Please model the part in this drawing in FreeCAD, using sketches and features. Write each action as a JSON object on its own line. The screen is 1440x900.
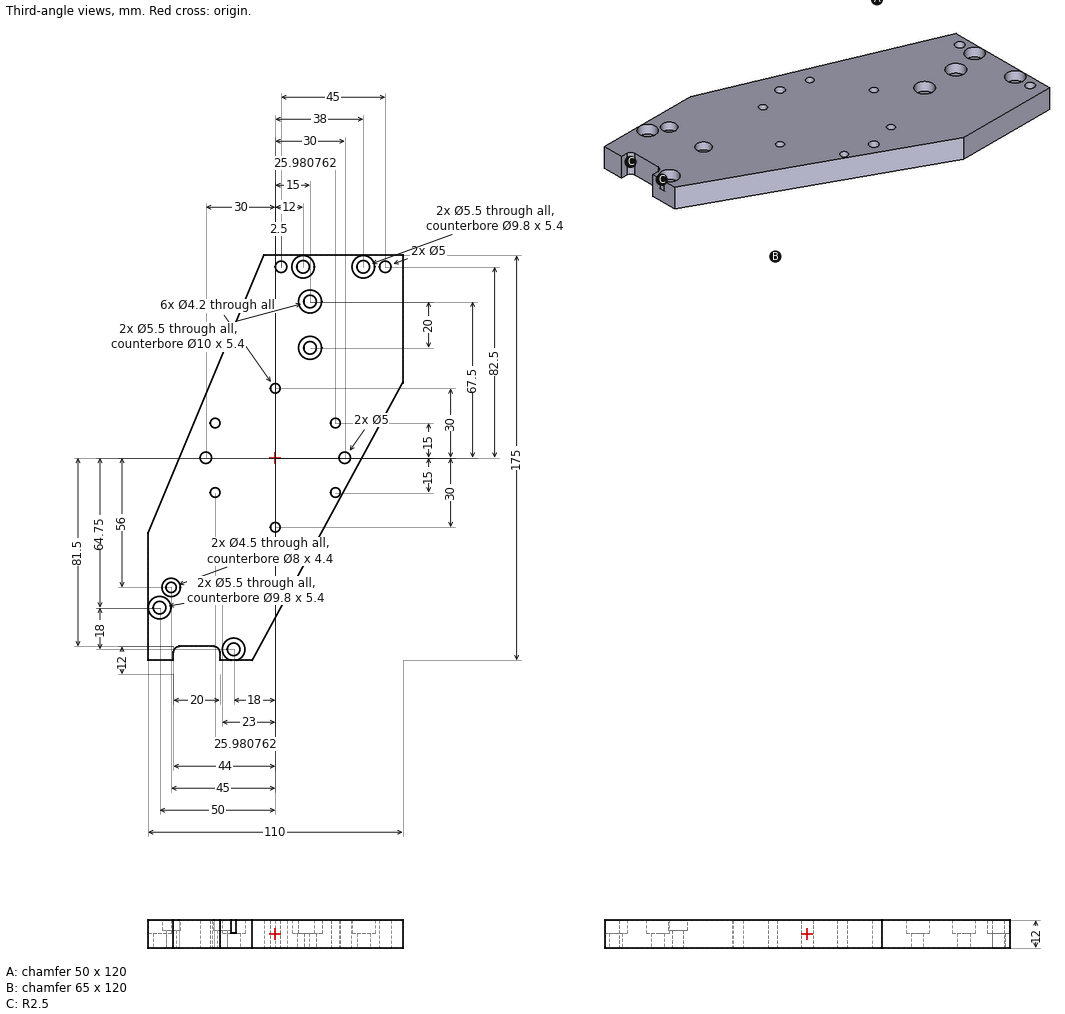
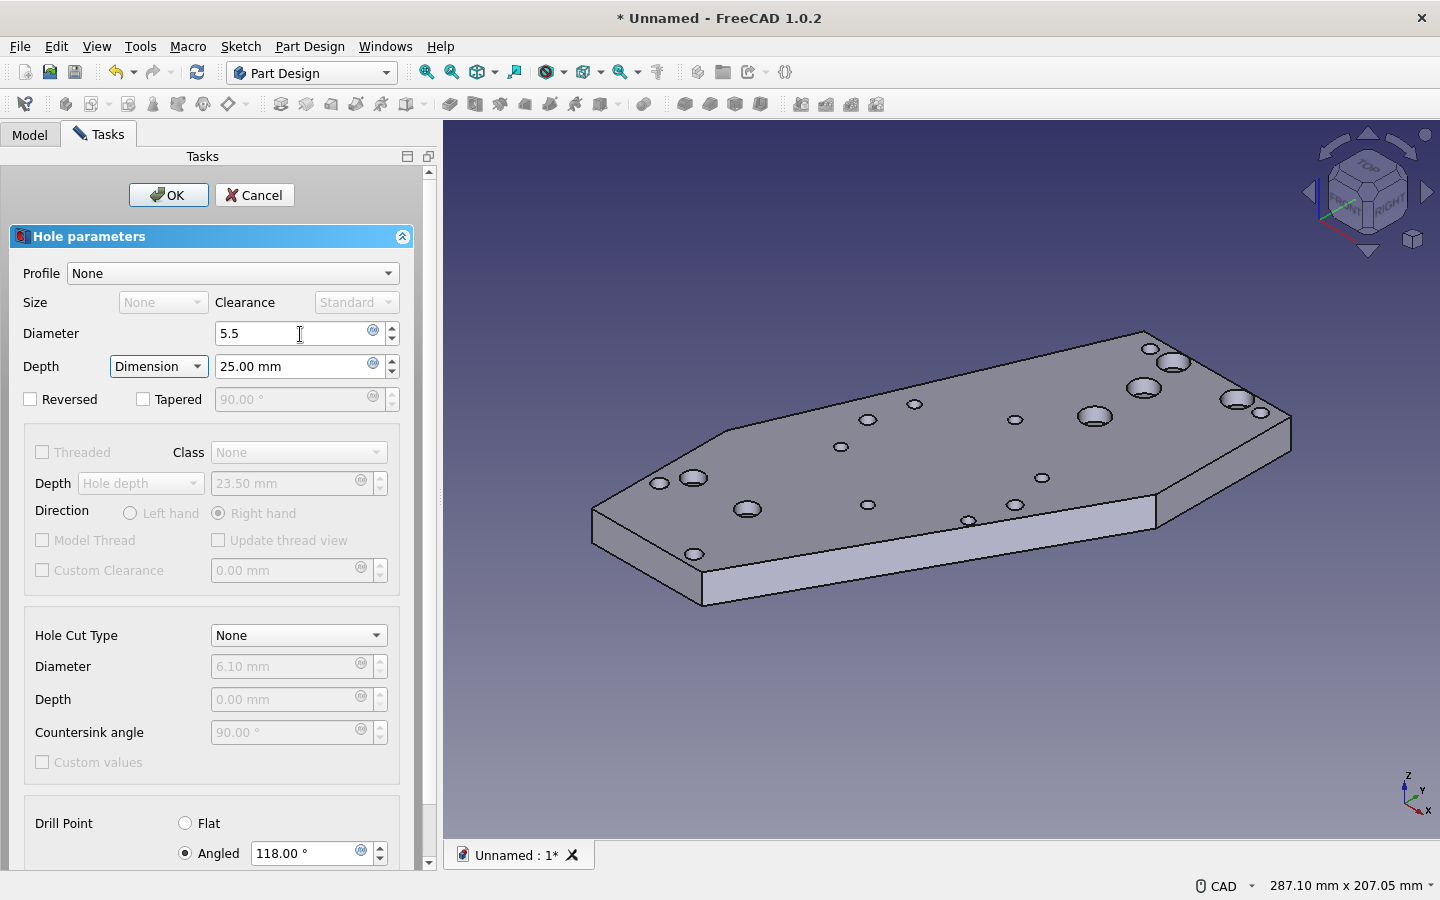
{"action": "left_click", "coordinate": [160, 366]}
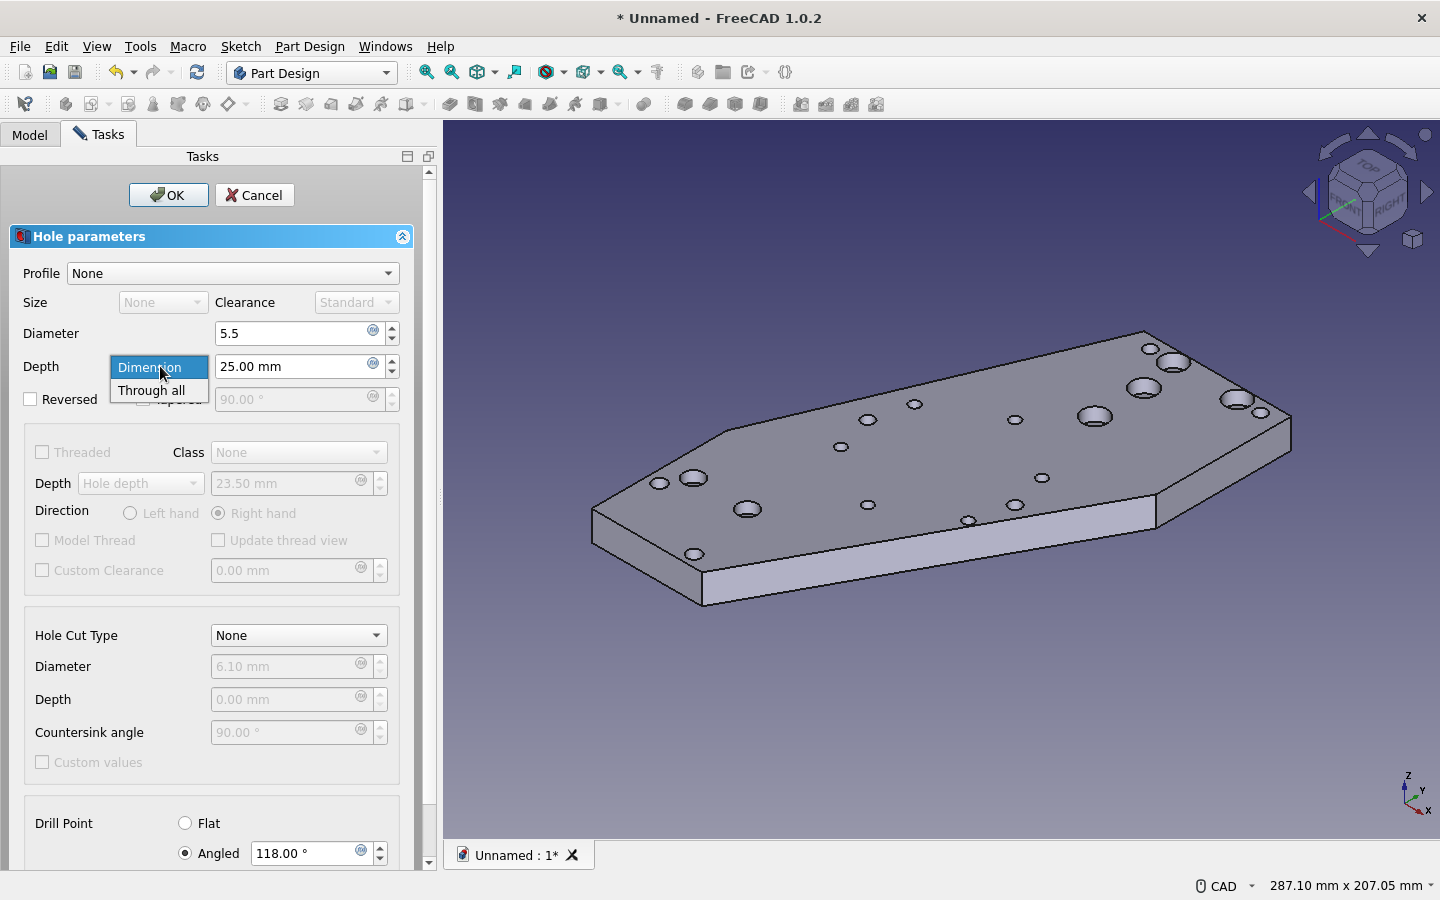
{"action": "left_click", "coordinate": [158, 390]}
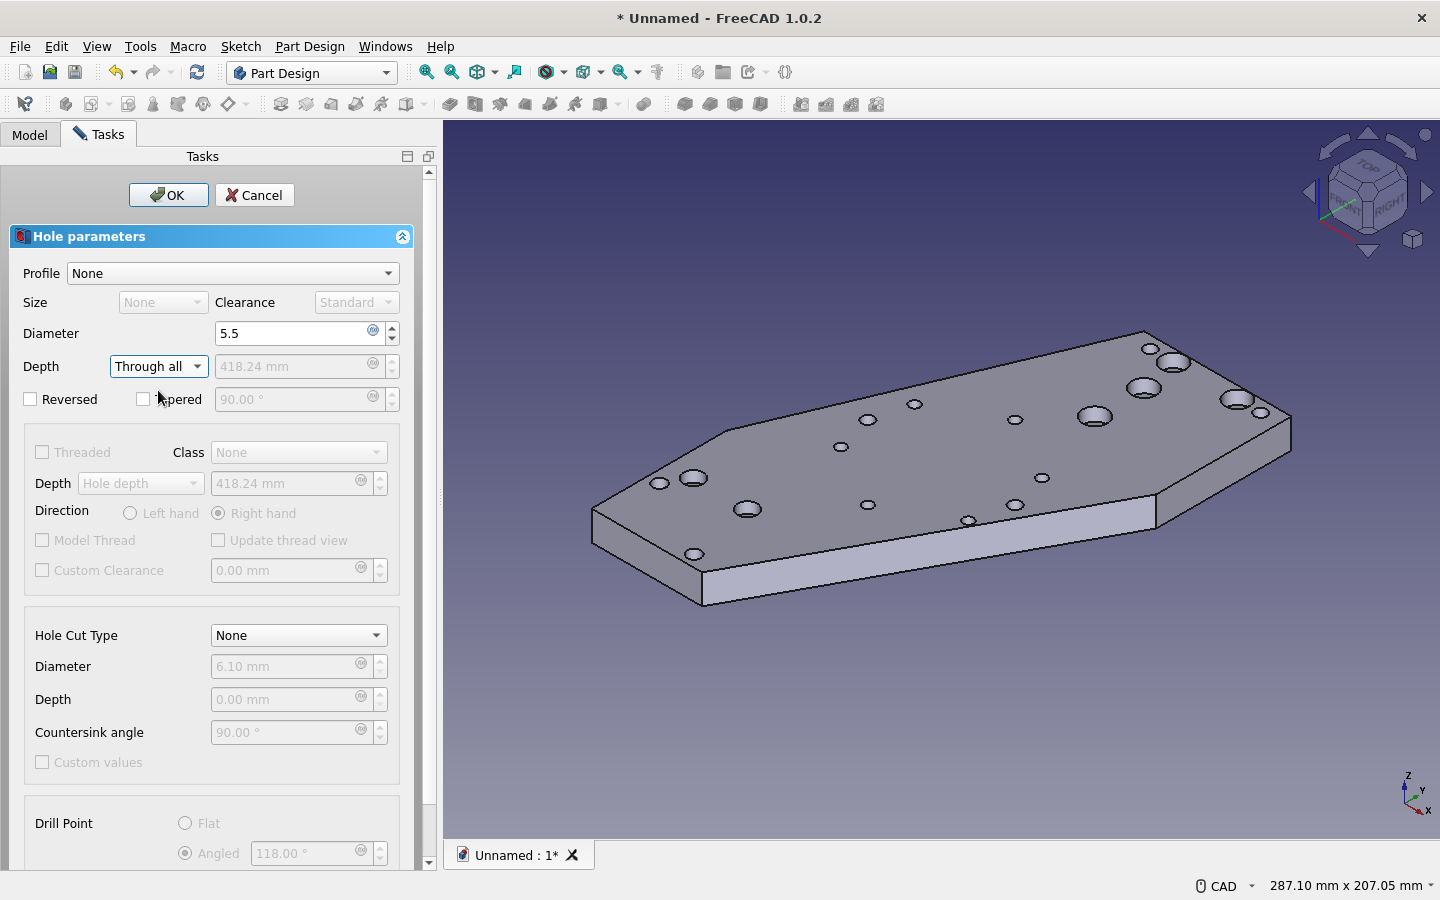
{"action": "left_click", "coordinate": [300, 636]}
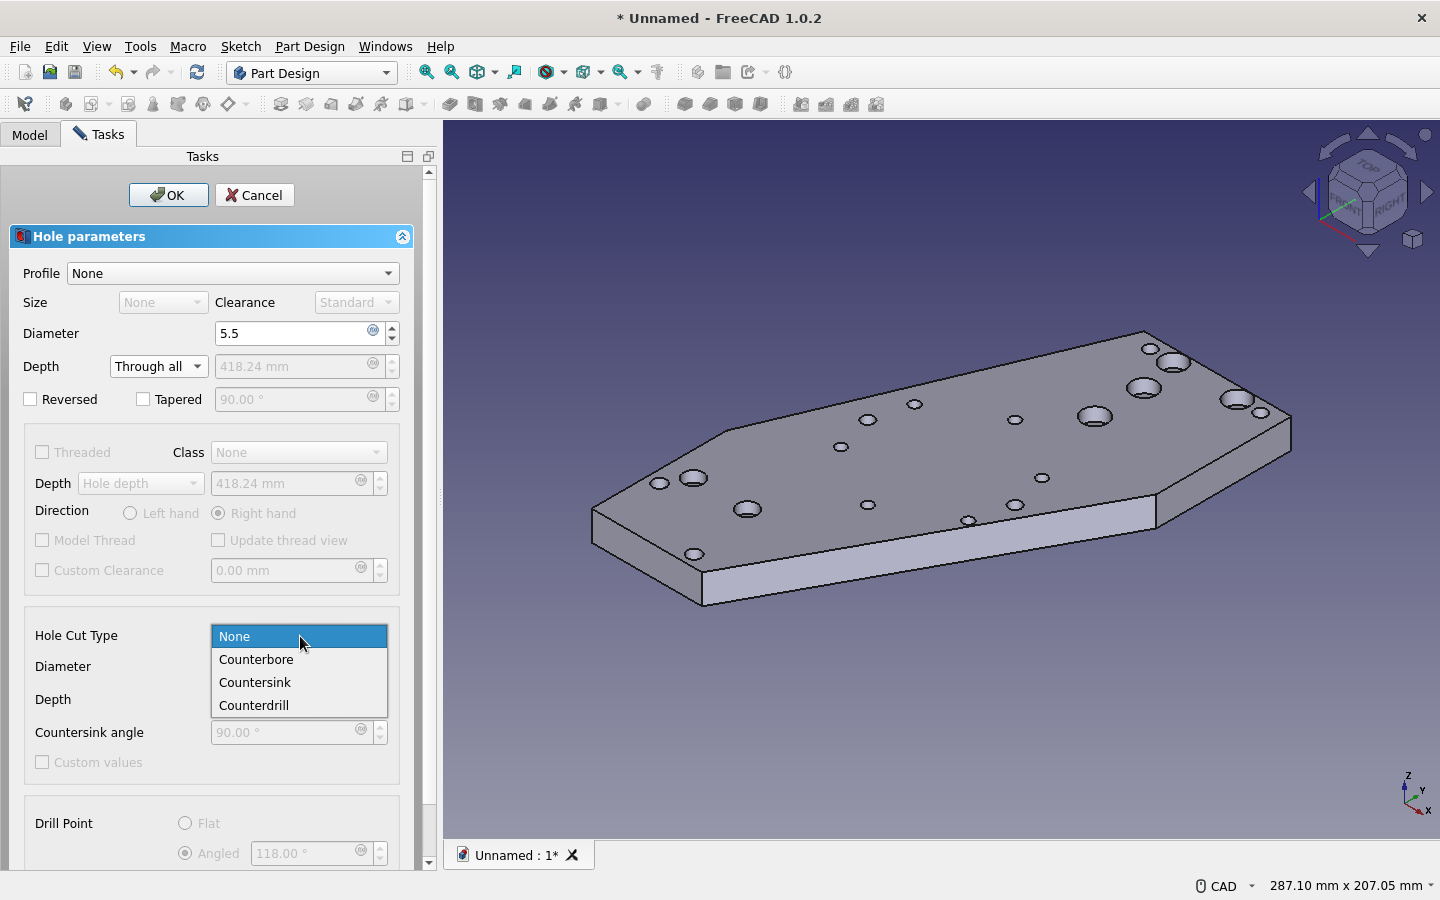
{"action": "left_click", "coordinate": [298, 660]}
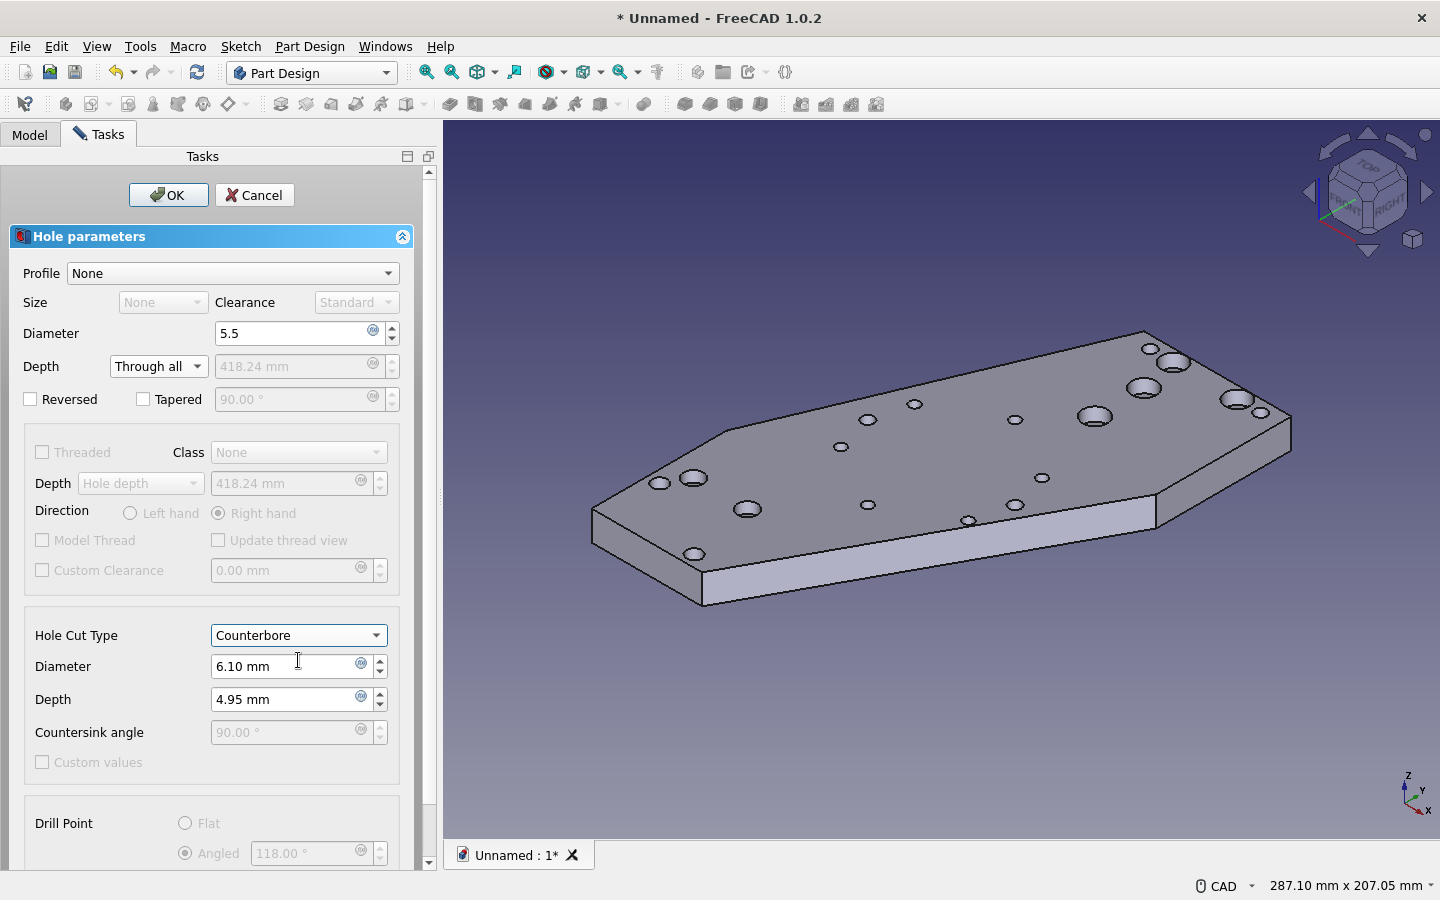
{"action": "triple_click", "coordinate": [292, 666]}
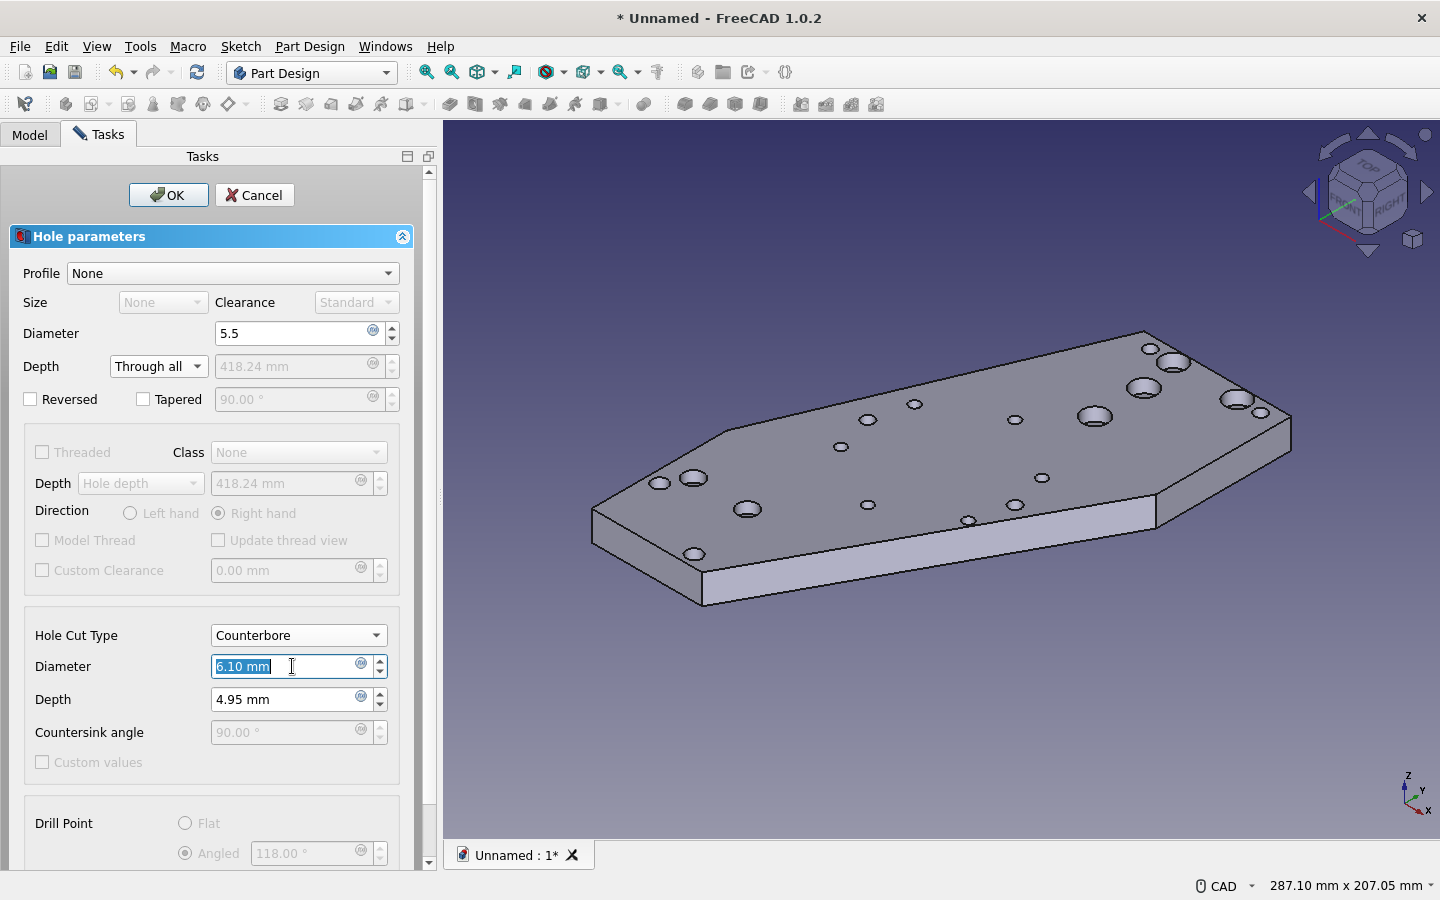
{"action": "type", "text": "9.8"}
{"action": "key", "text": "Tab"}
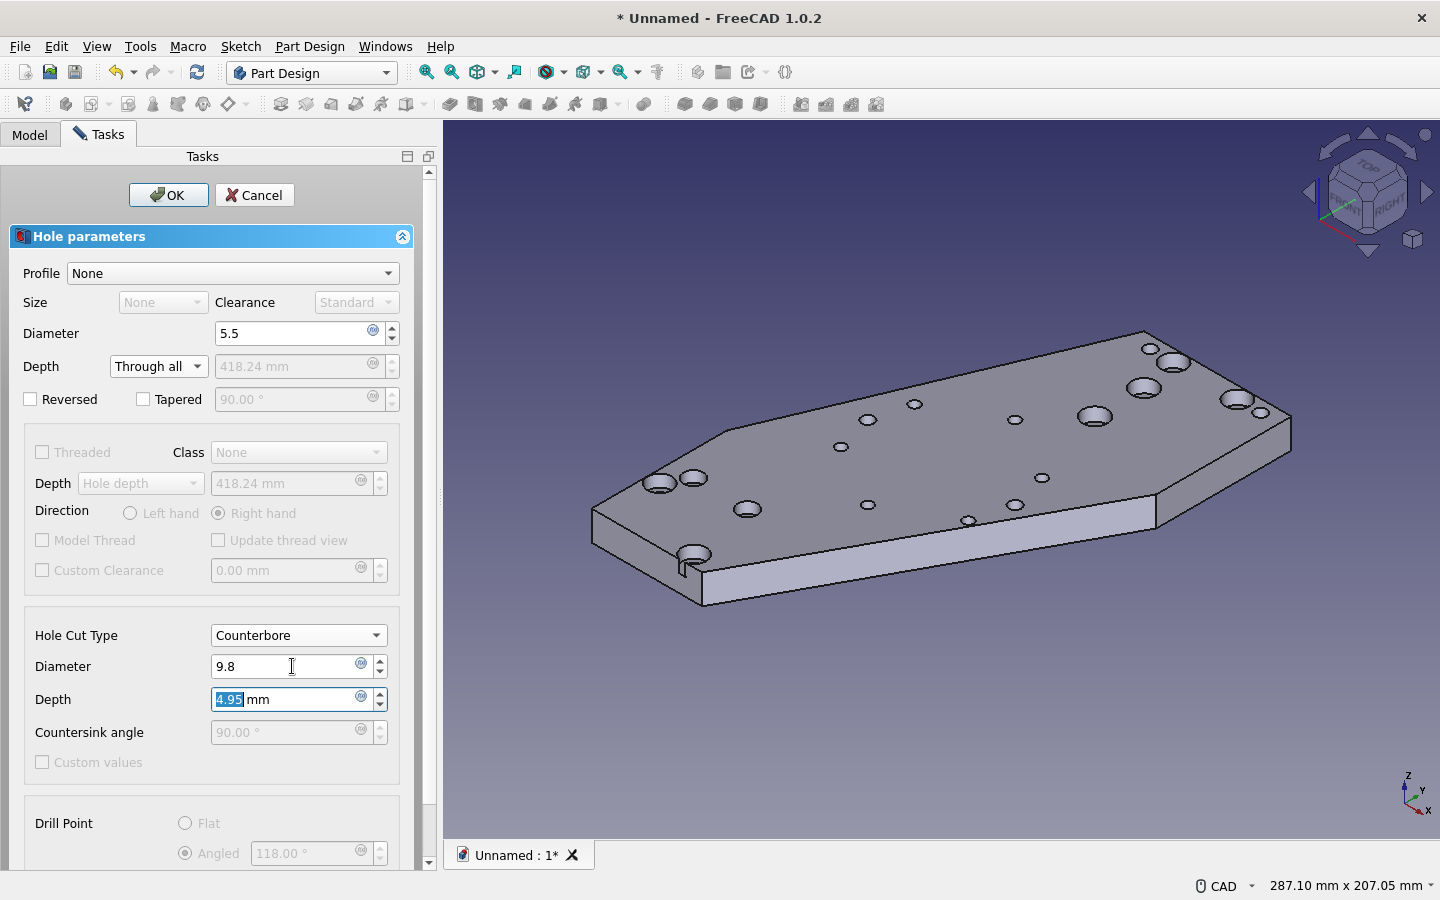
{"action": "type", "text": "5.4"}
{"action": "key", "text": "Tab"}